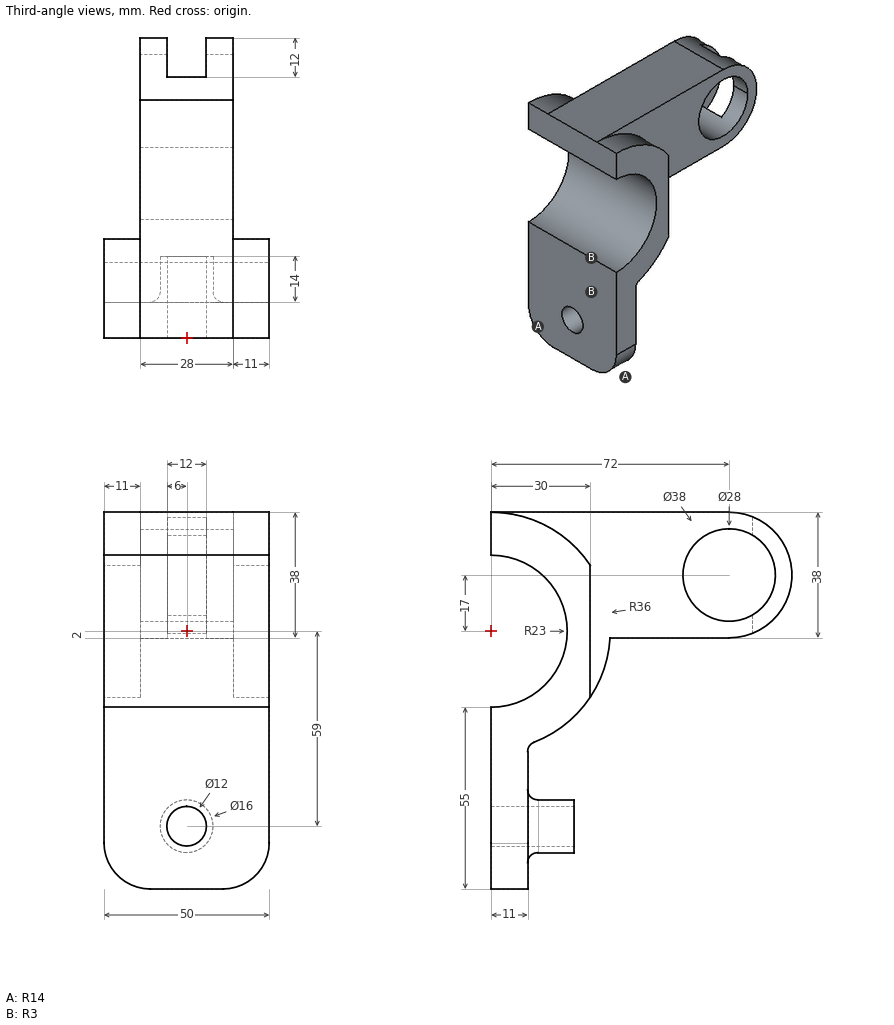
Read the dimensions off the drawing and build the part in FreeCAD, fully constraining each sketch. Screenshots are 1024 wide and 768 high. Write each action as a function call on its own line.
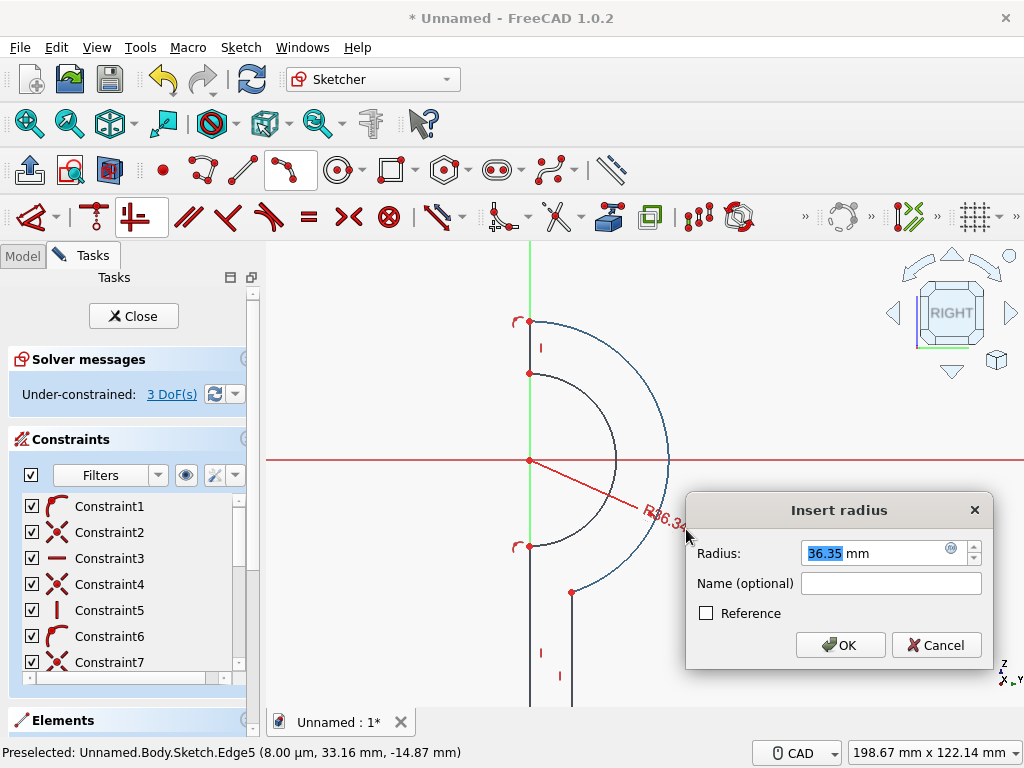
text(36)
key(Return)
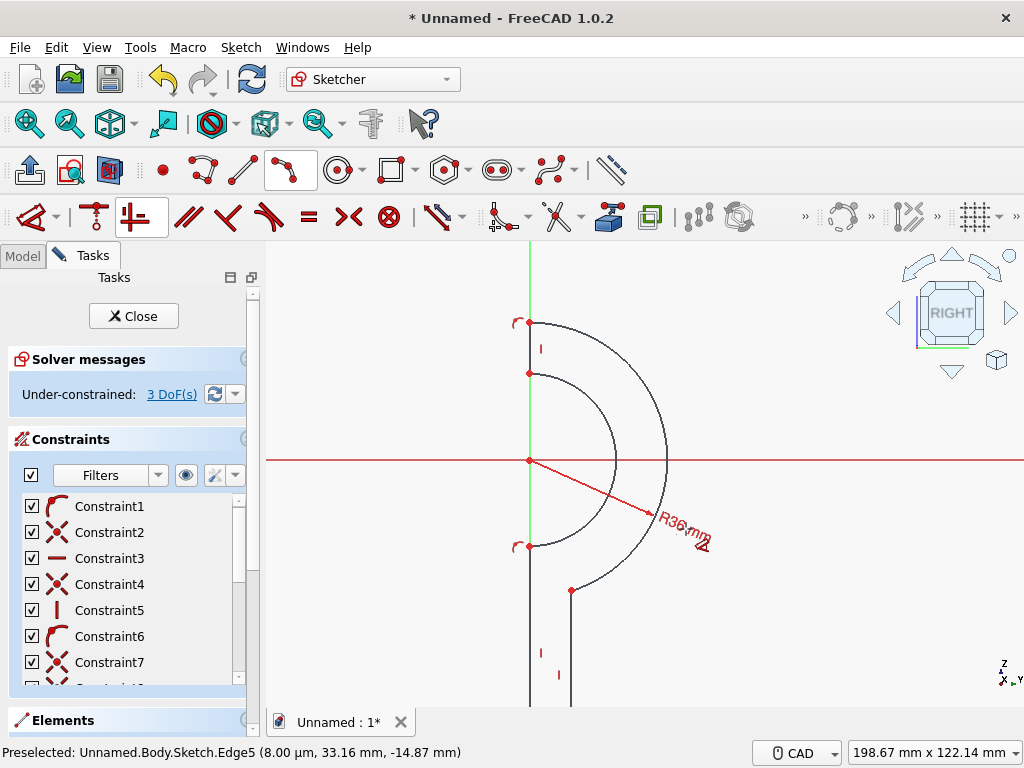
click(600, 511)
click(581, 567)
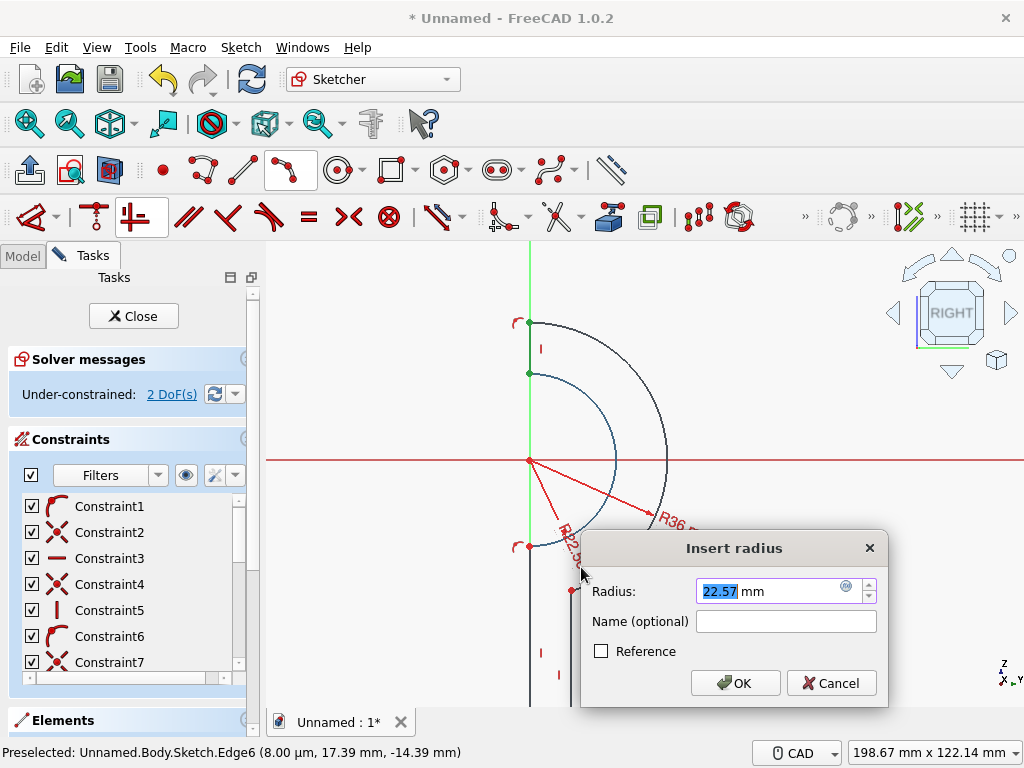
text(23)
key(Return)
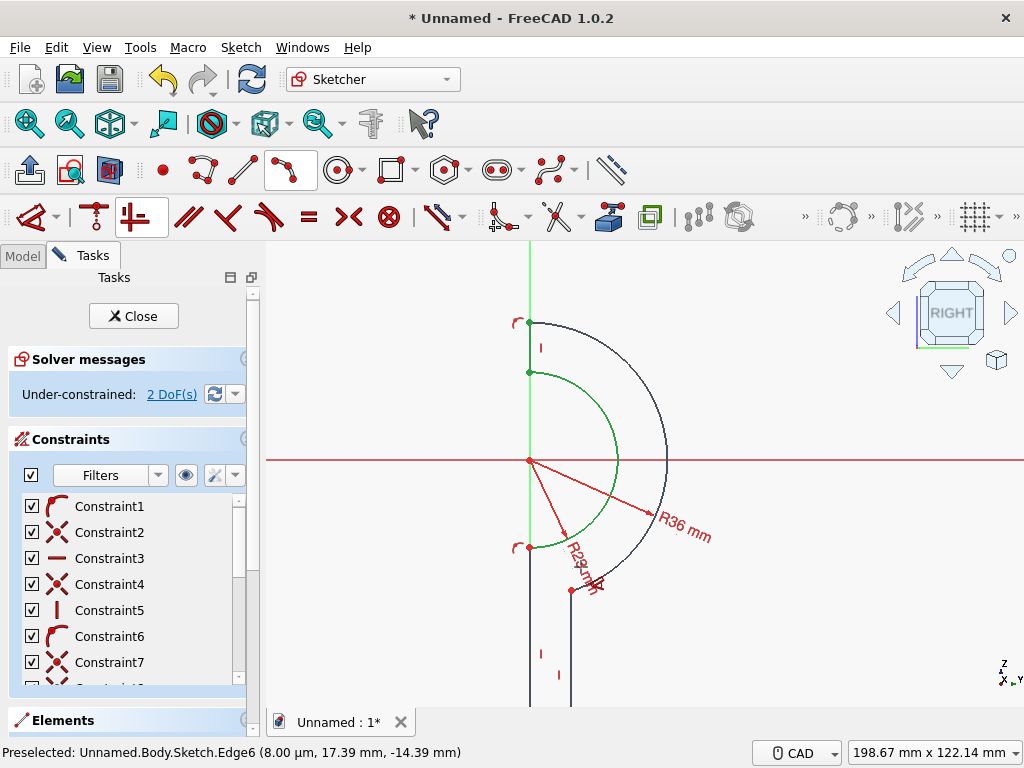
click(530, 611)
click(496, 613)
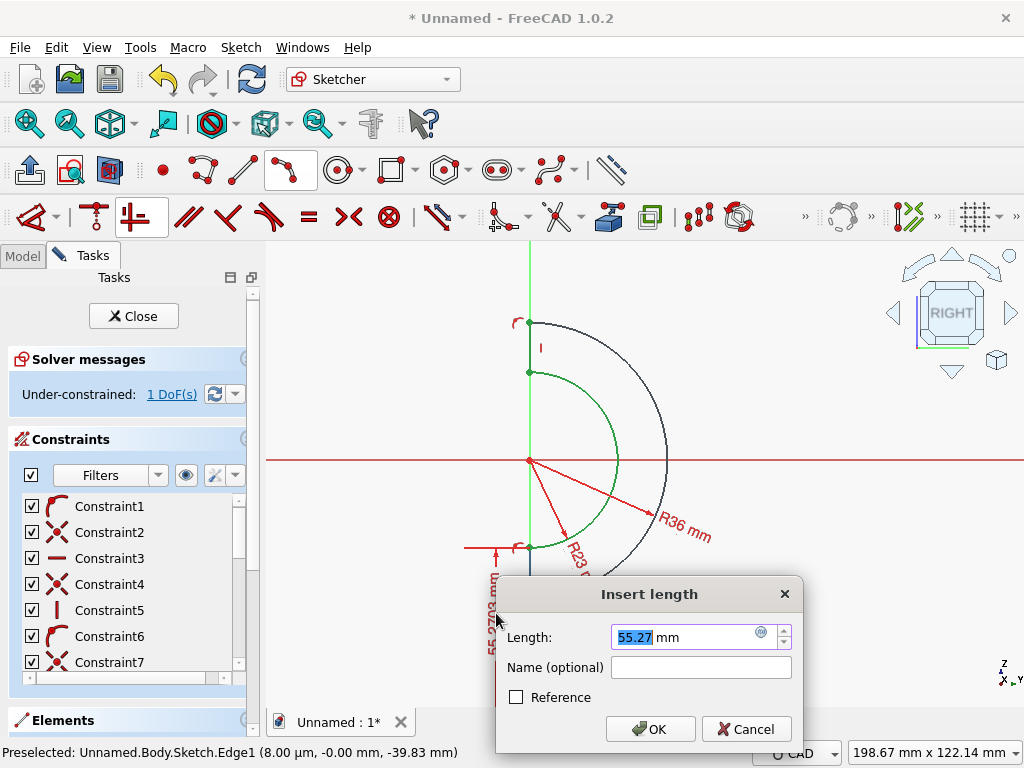
text(55)
key(Return)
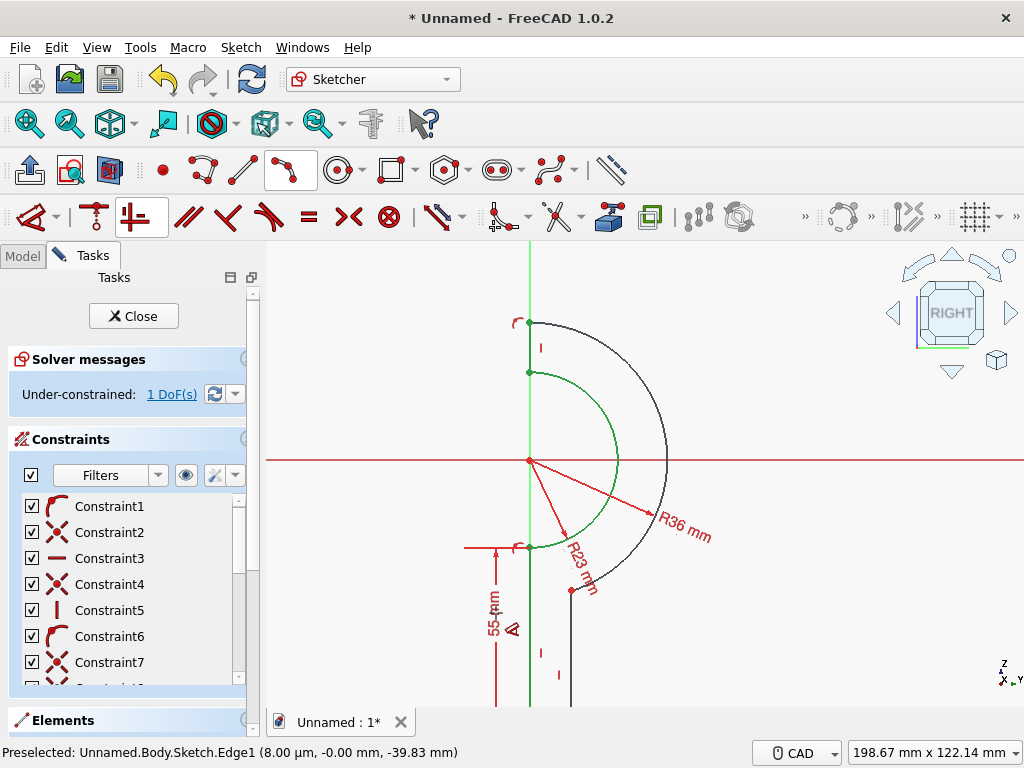
scroll(533, 339, down, 2)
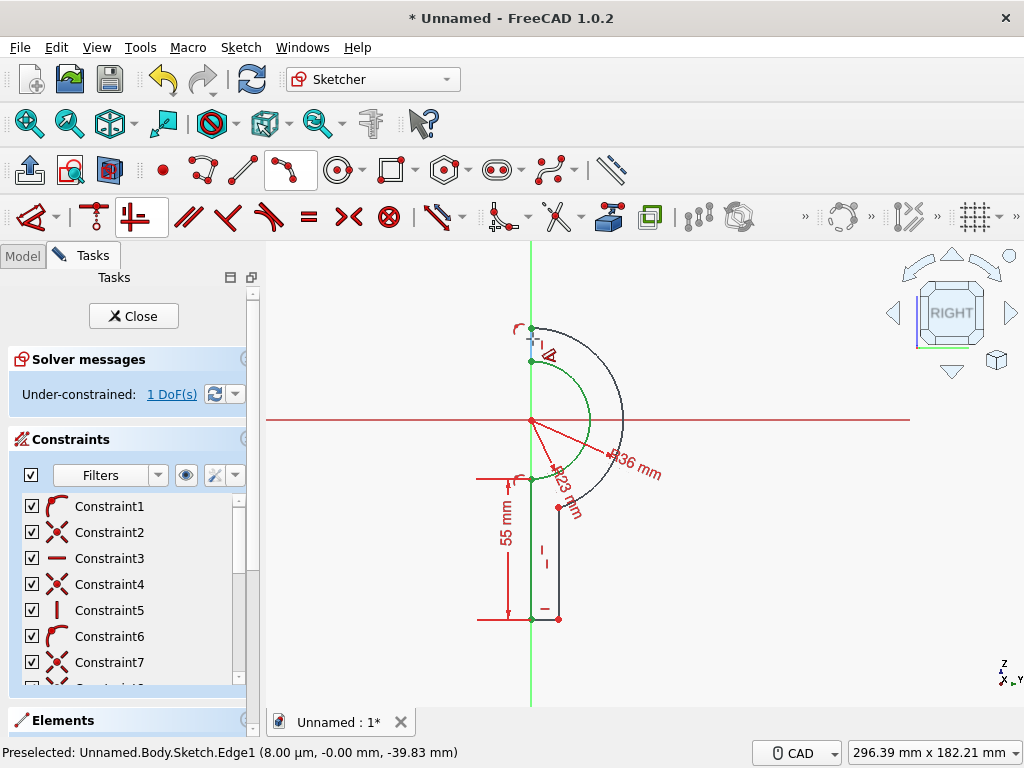
scroll(539, 620, up, 3)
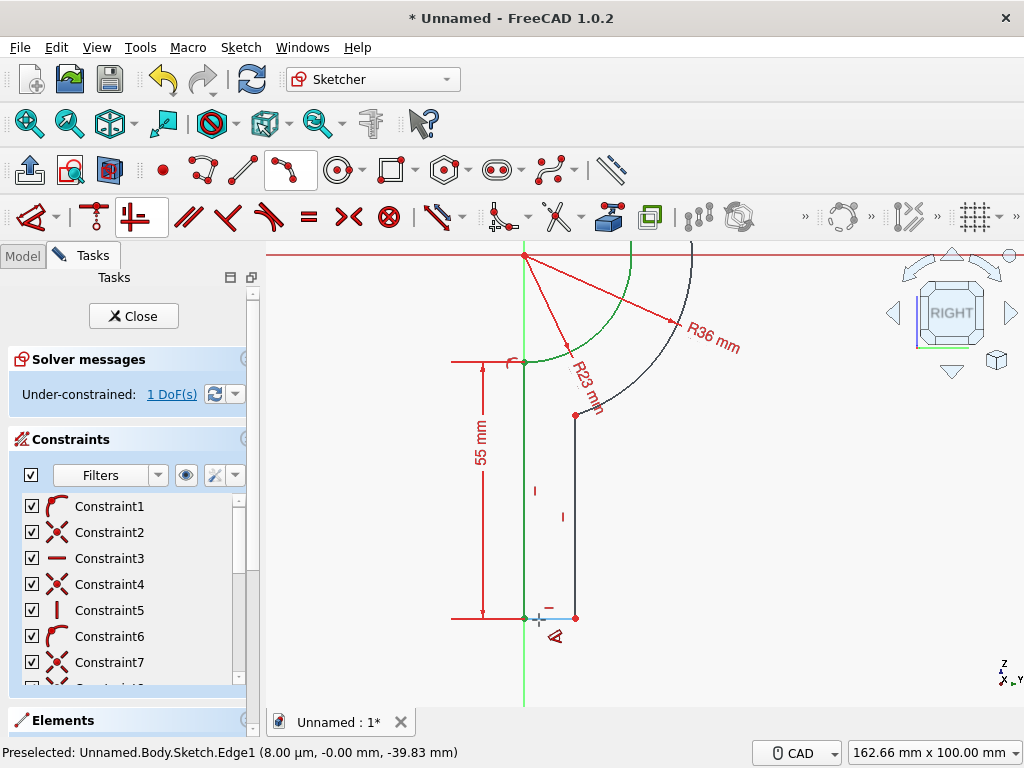
click(539, 619)
click(550, 653)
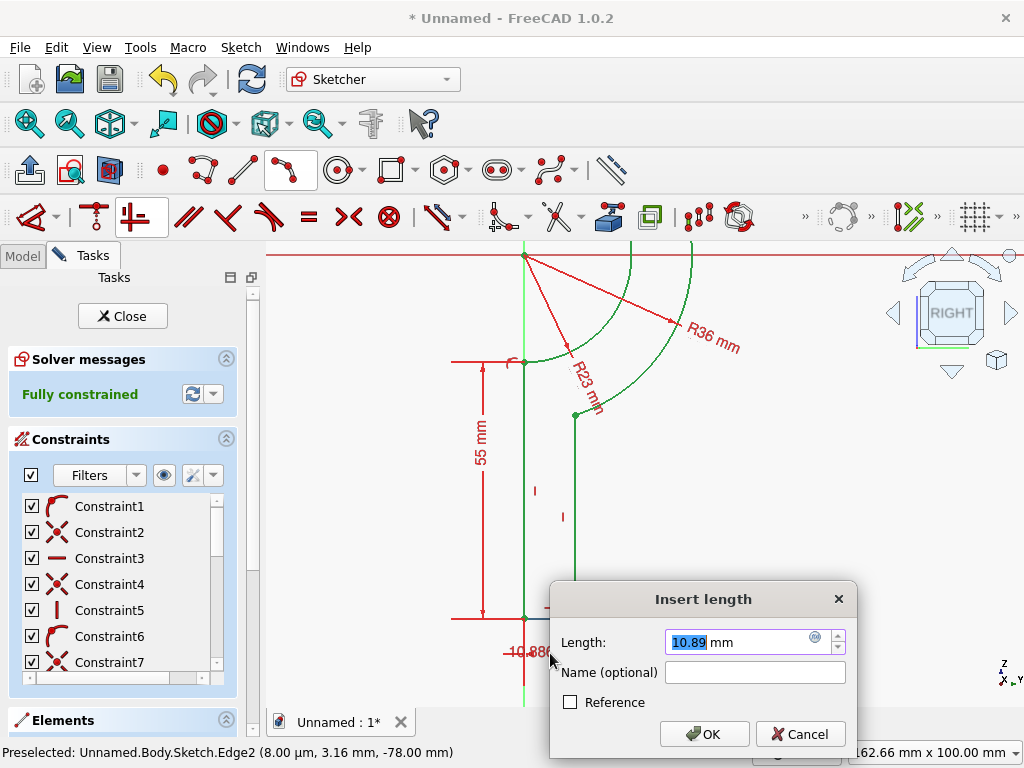
text(11)
key(Return)
key(Escape)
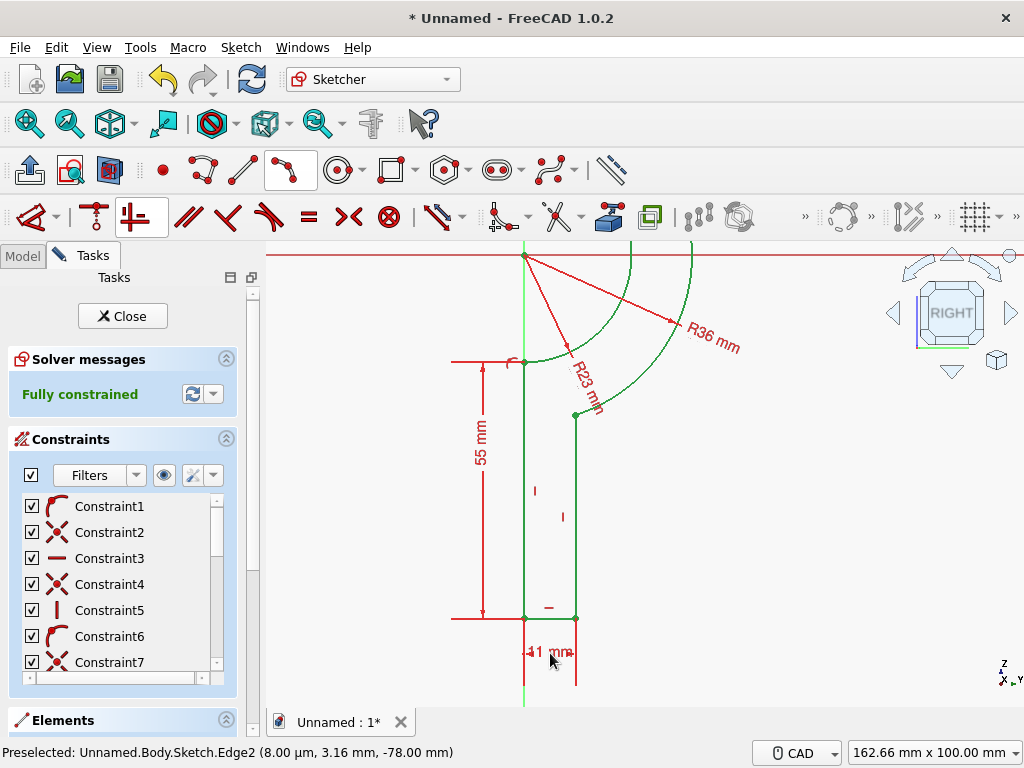
click(123, 316)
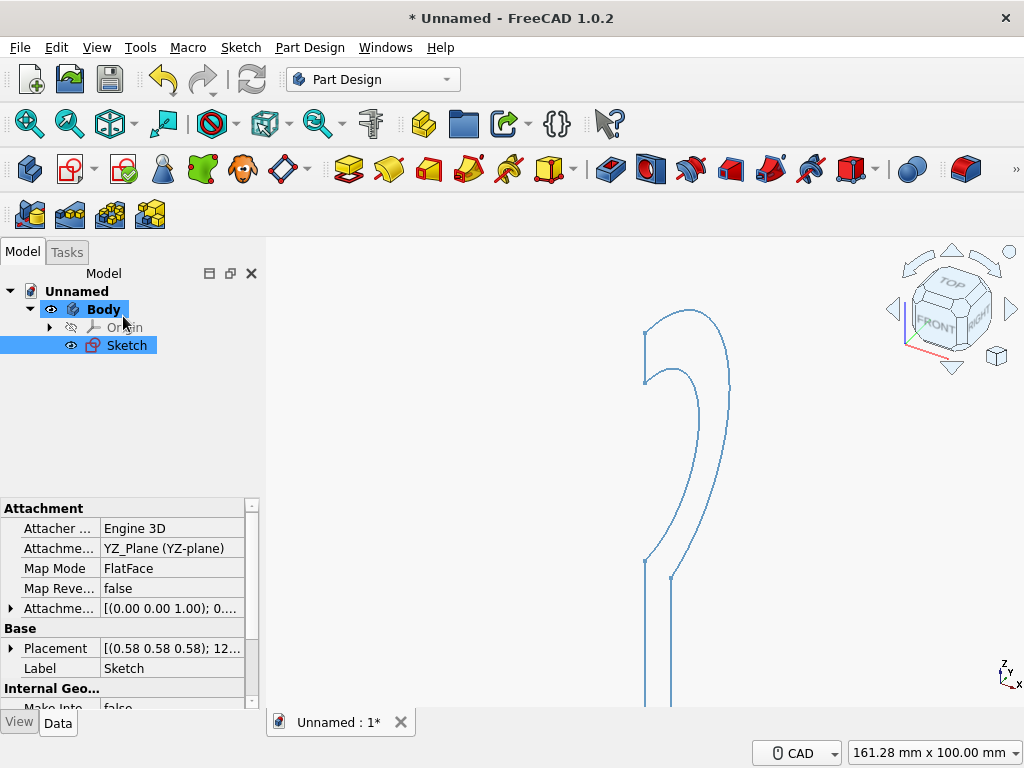
click(350, 170)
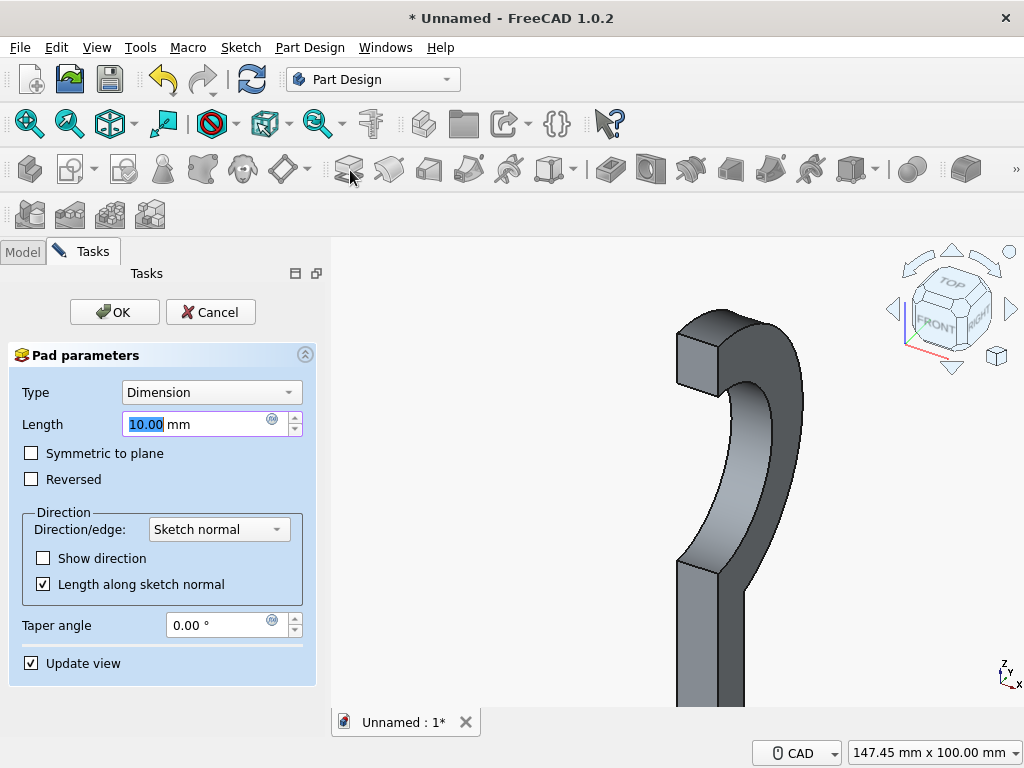
text(50)
key(Tab)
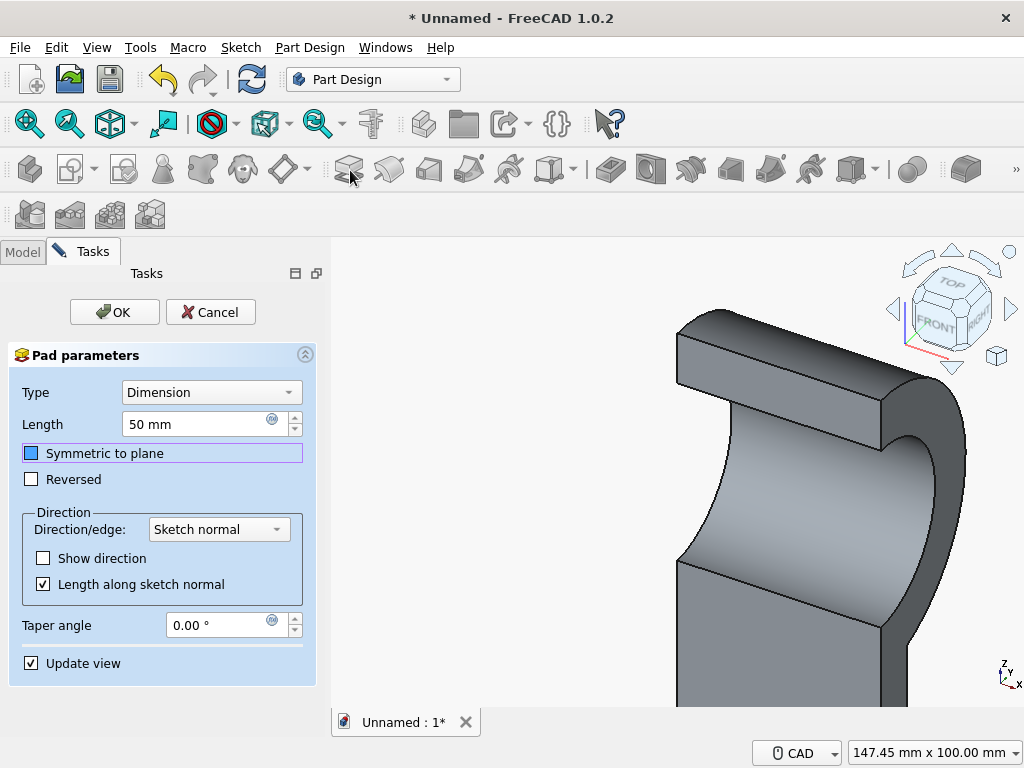
click(30, 453)